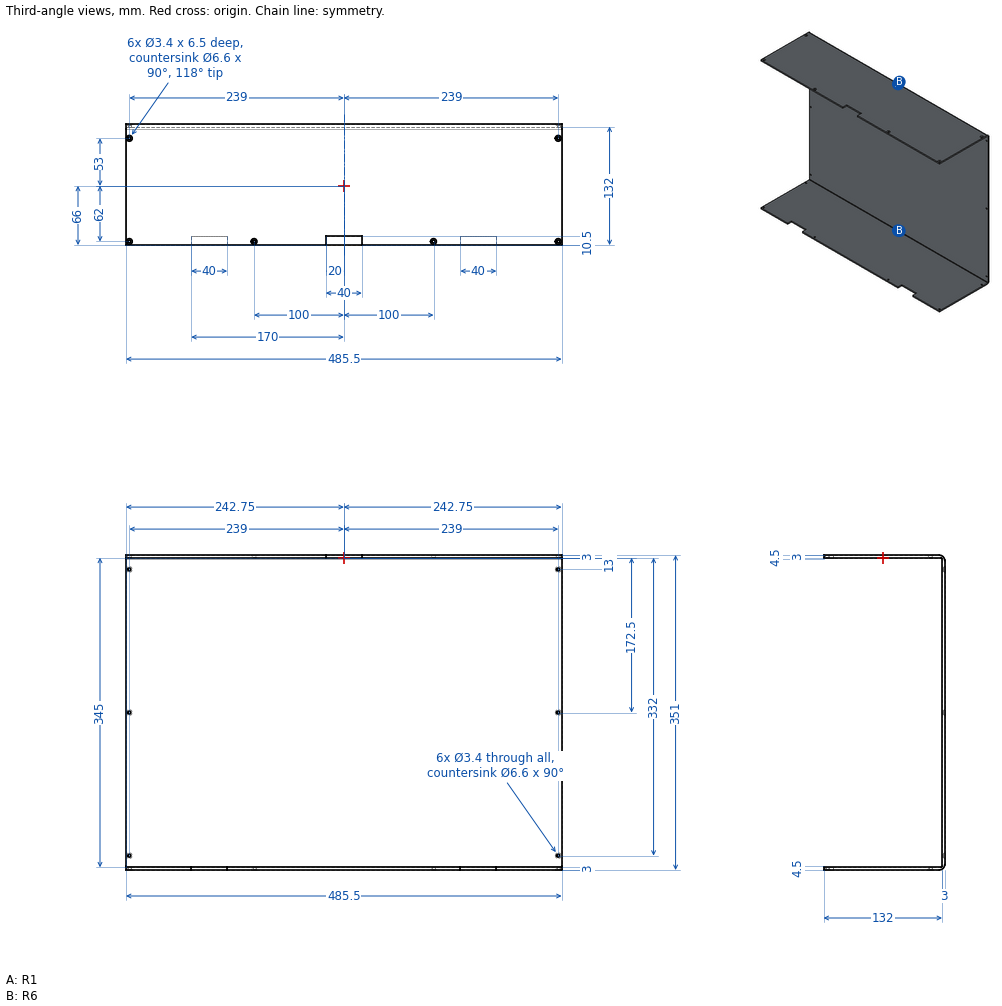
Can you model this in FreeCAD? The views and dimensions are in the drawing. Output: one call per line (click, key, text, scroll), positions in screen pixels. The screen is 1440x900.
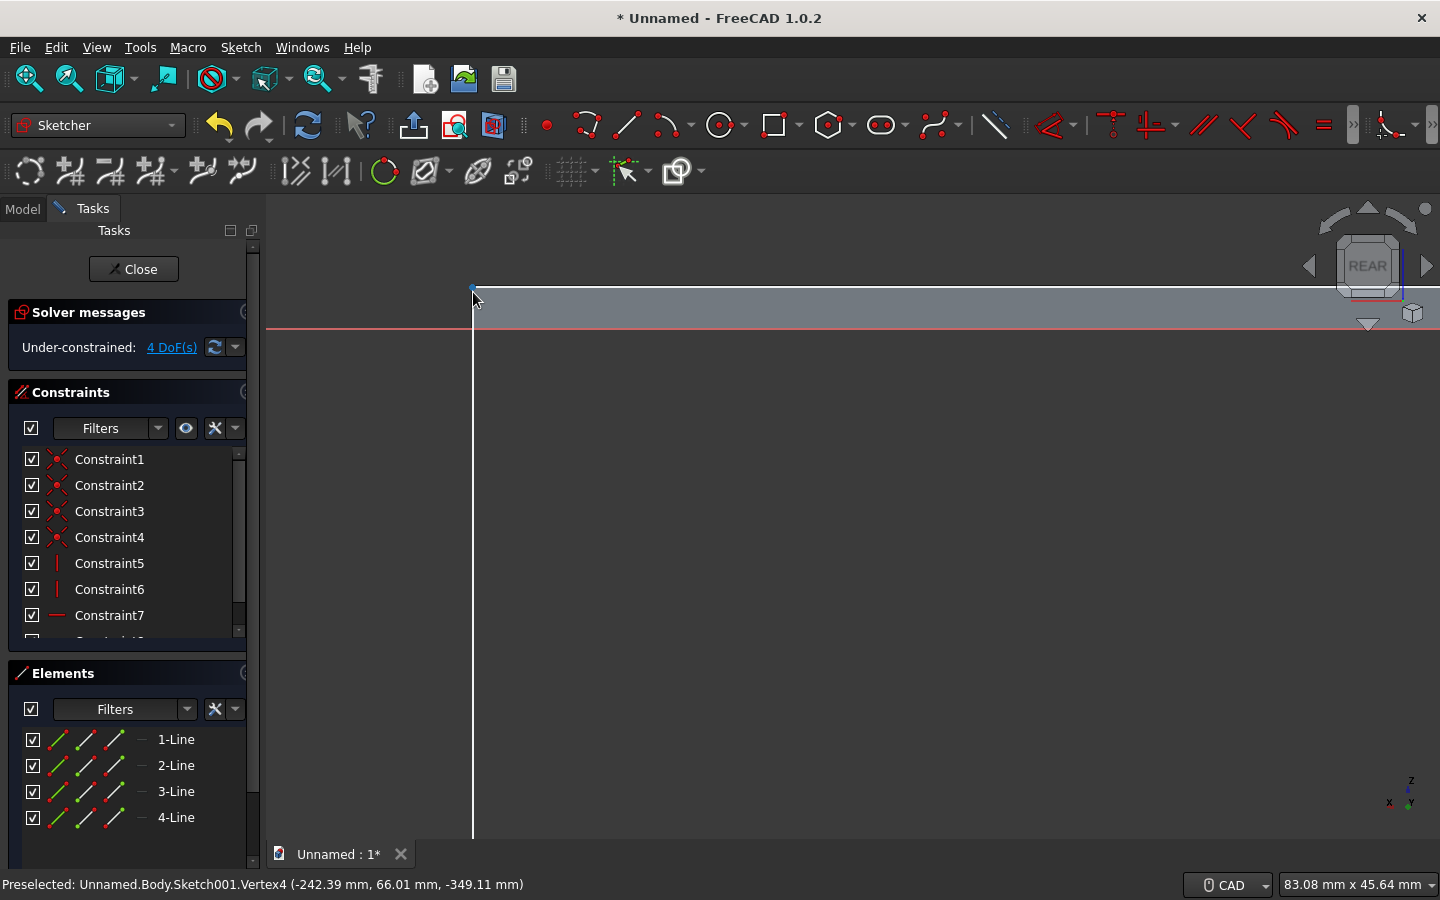
click(473, 287)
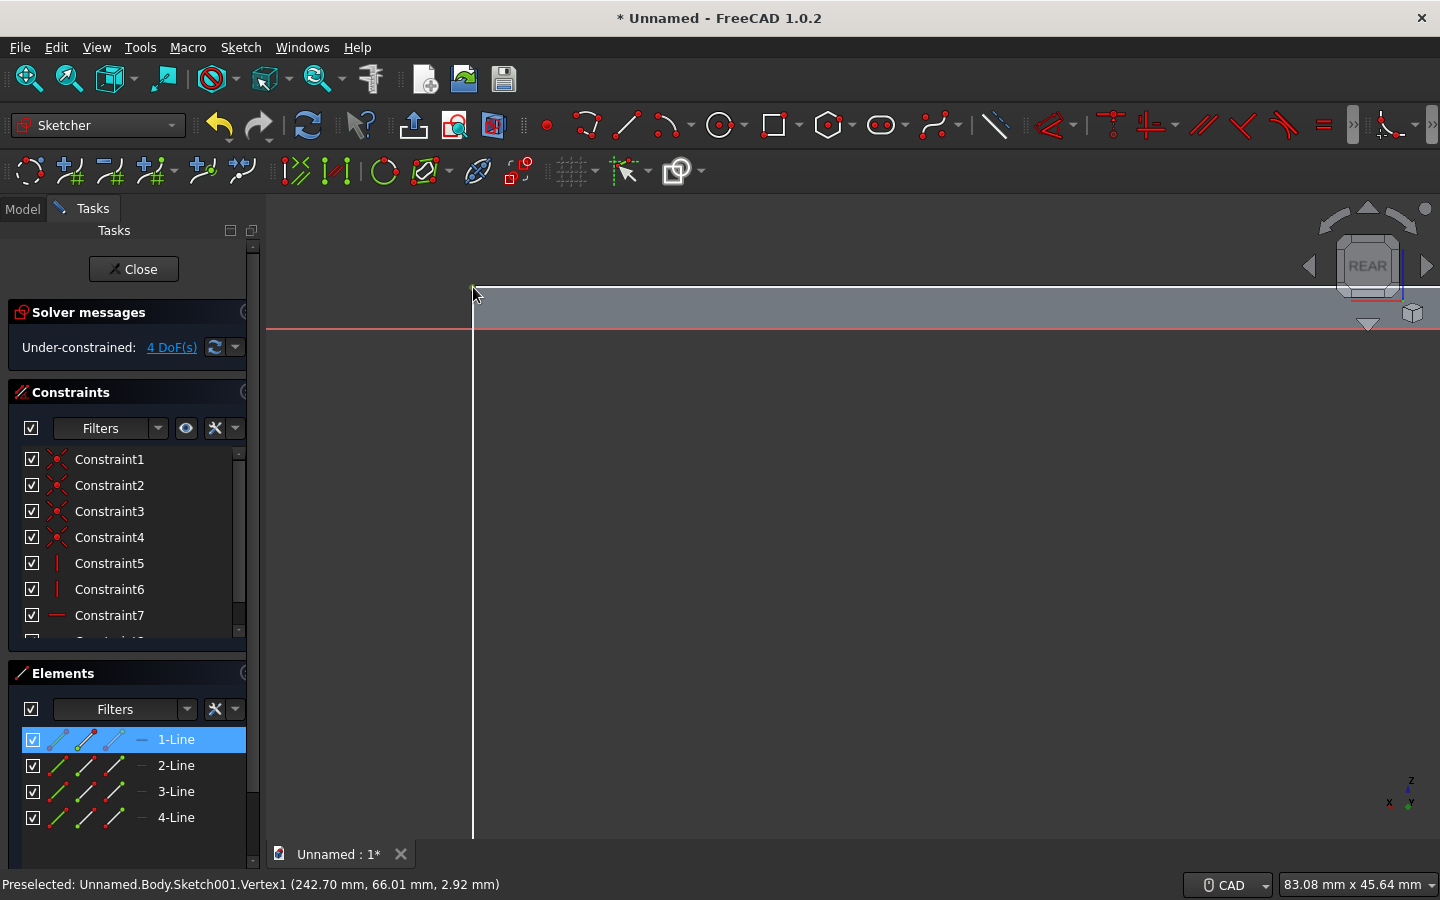
key(i)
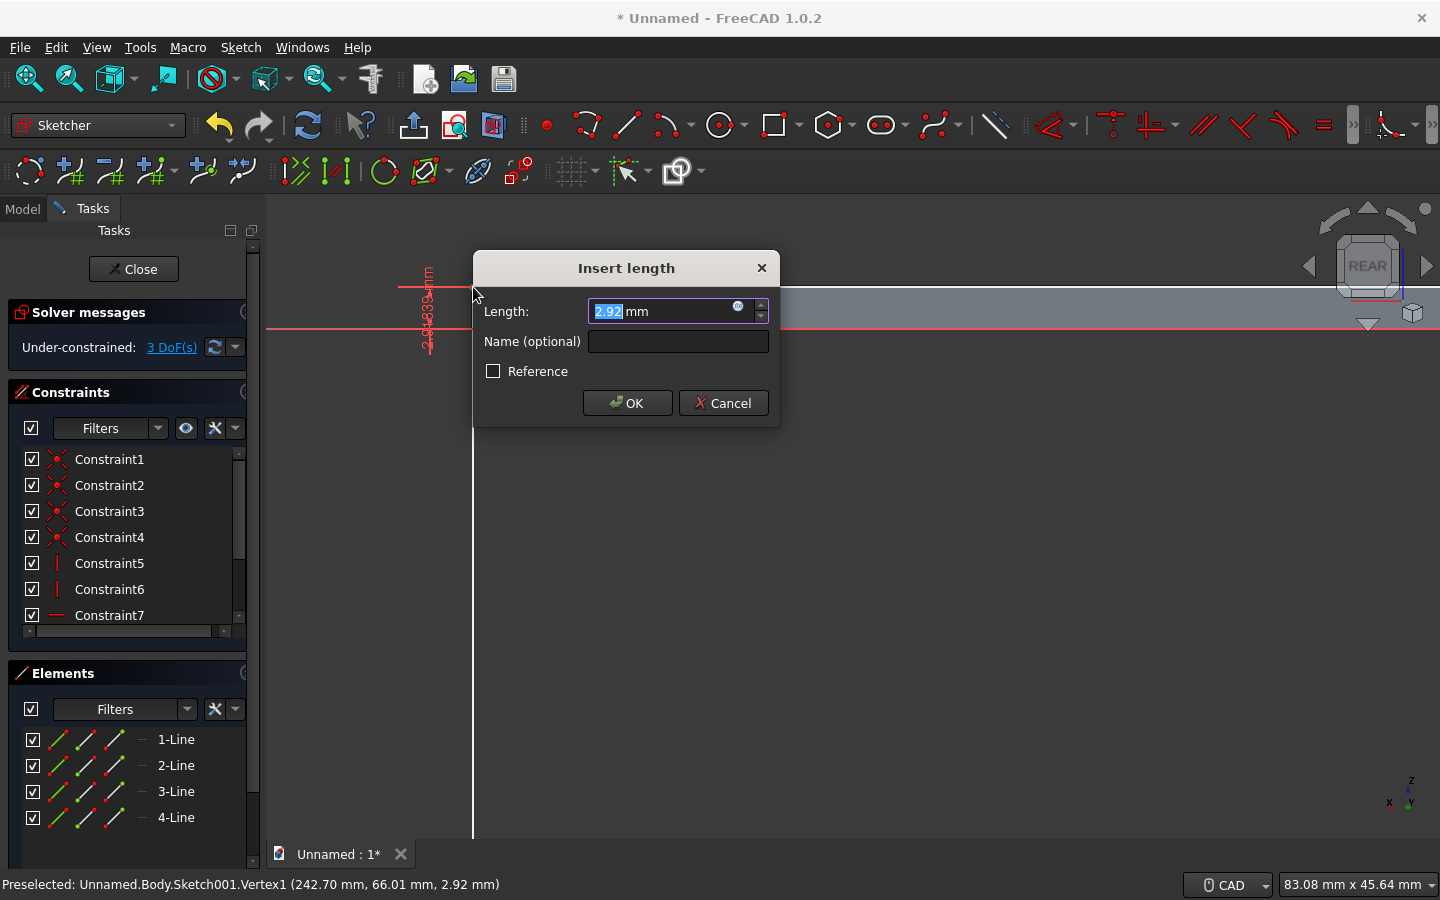
text(3)
key(Return)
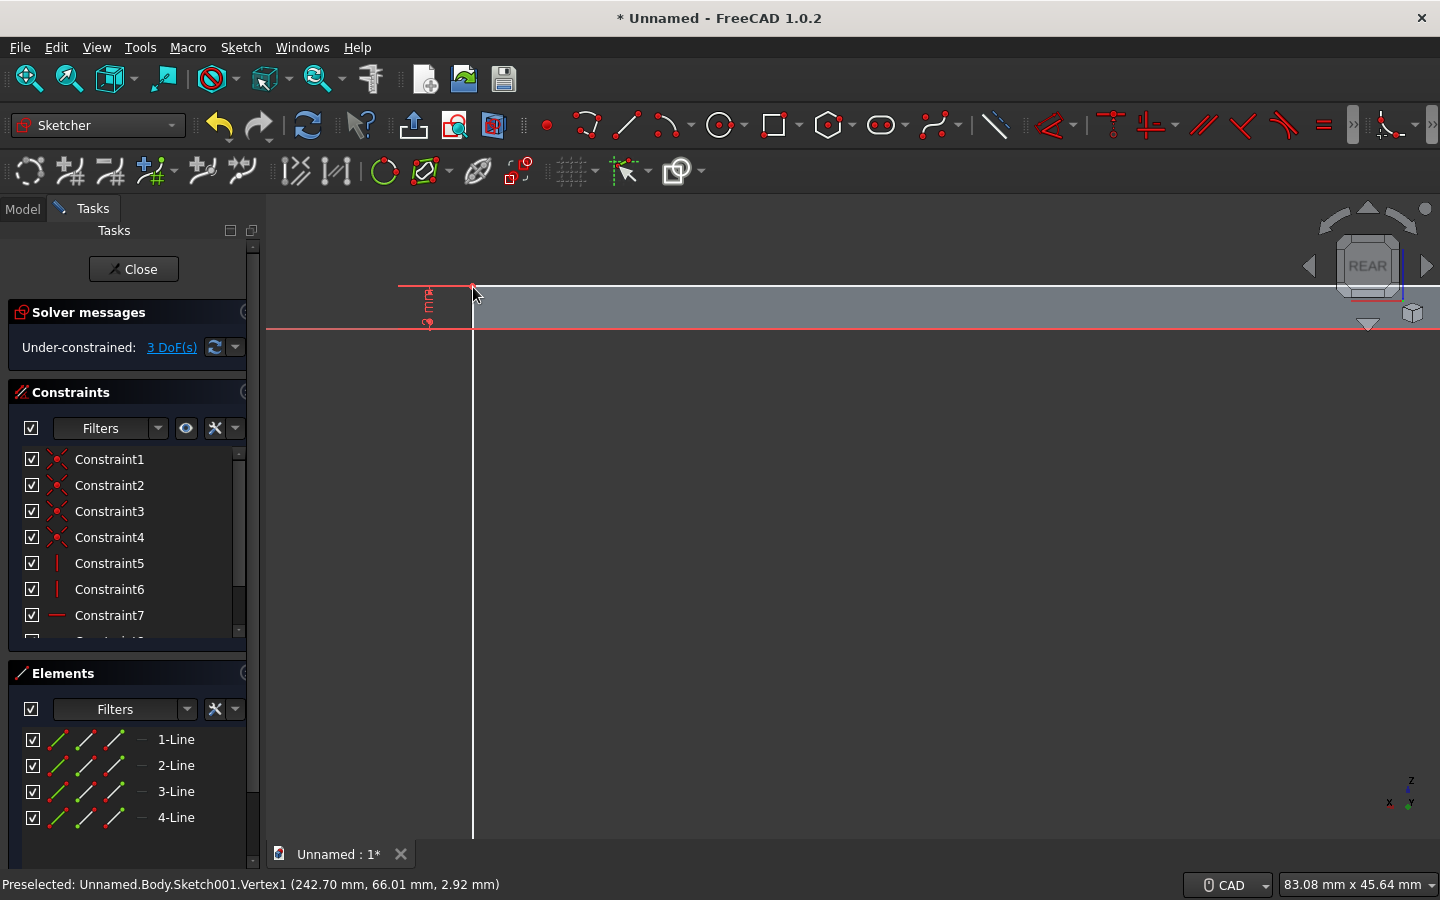
scroll(473, 292, down, 12)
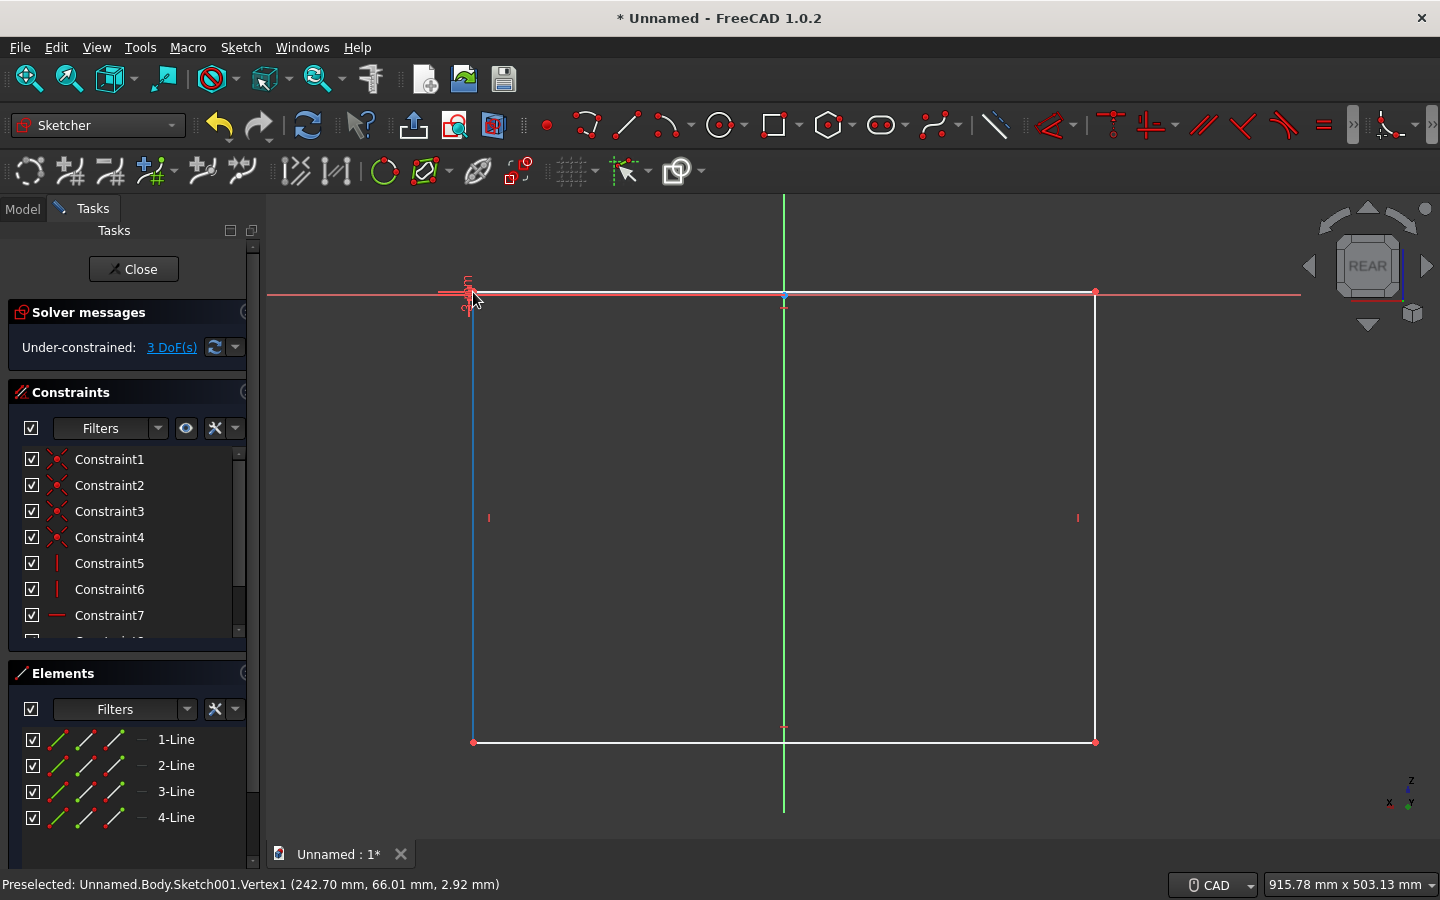
click(473, 427)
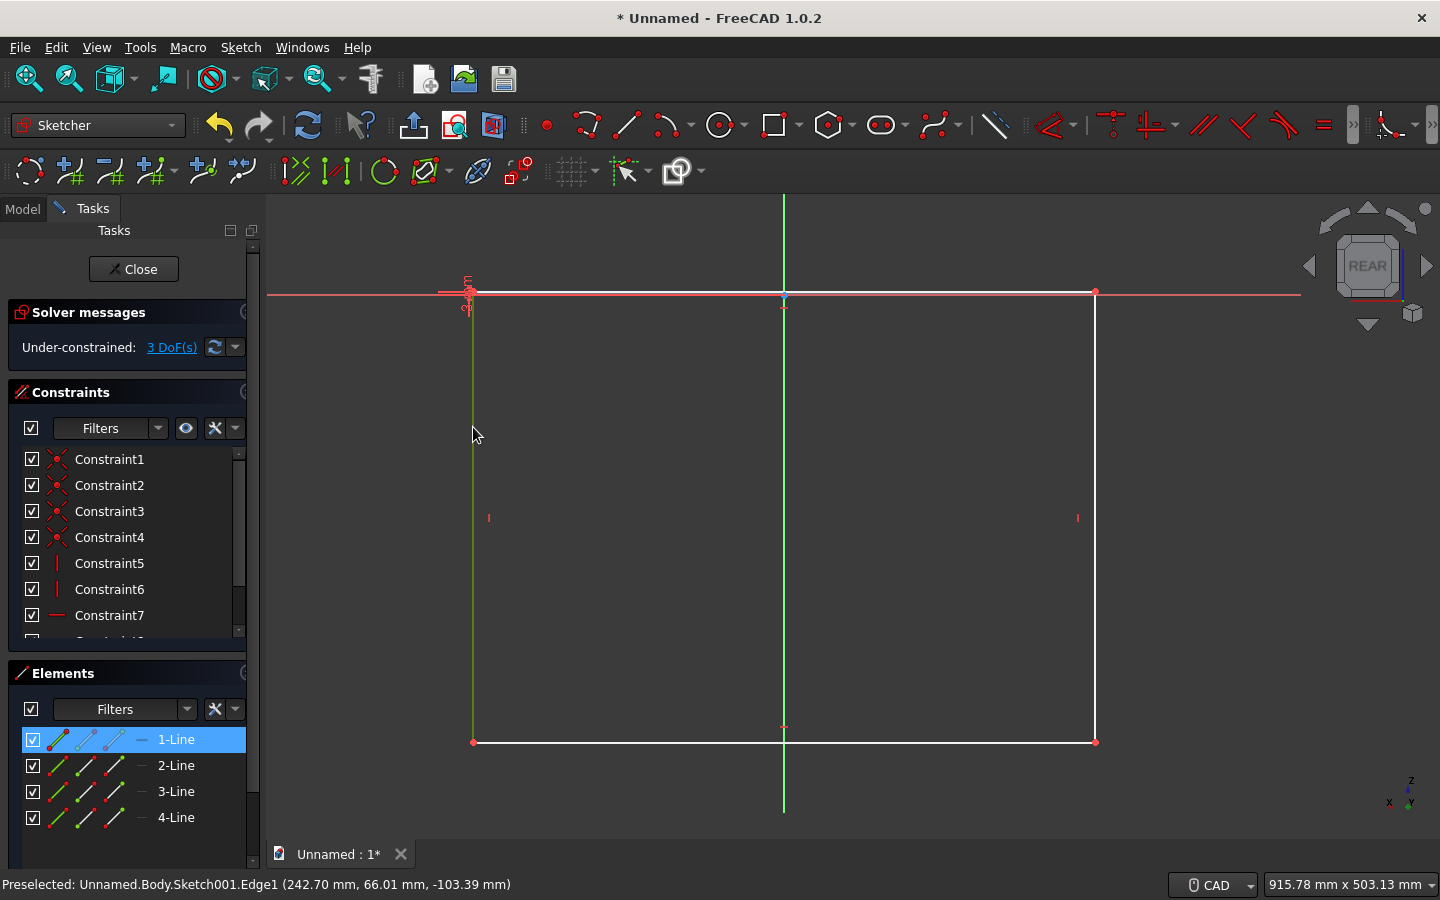
key(i)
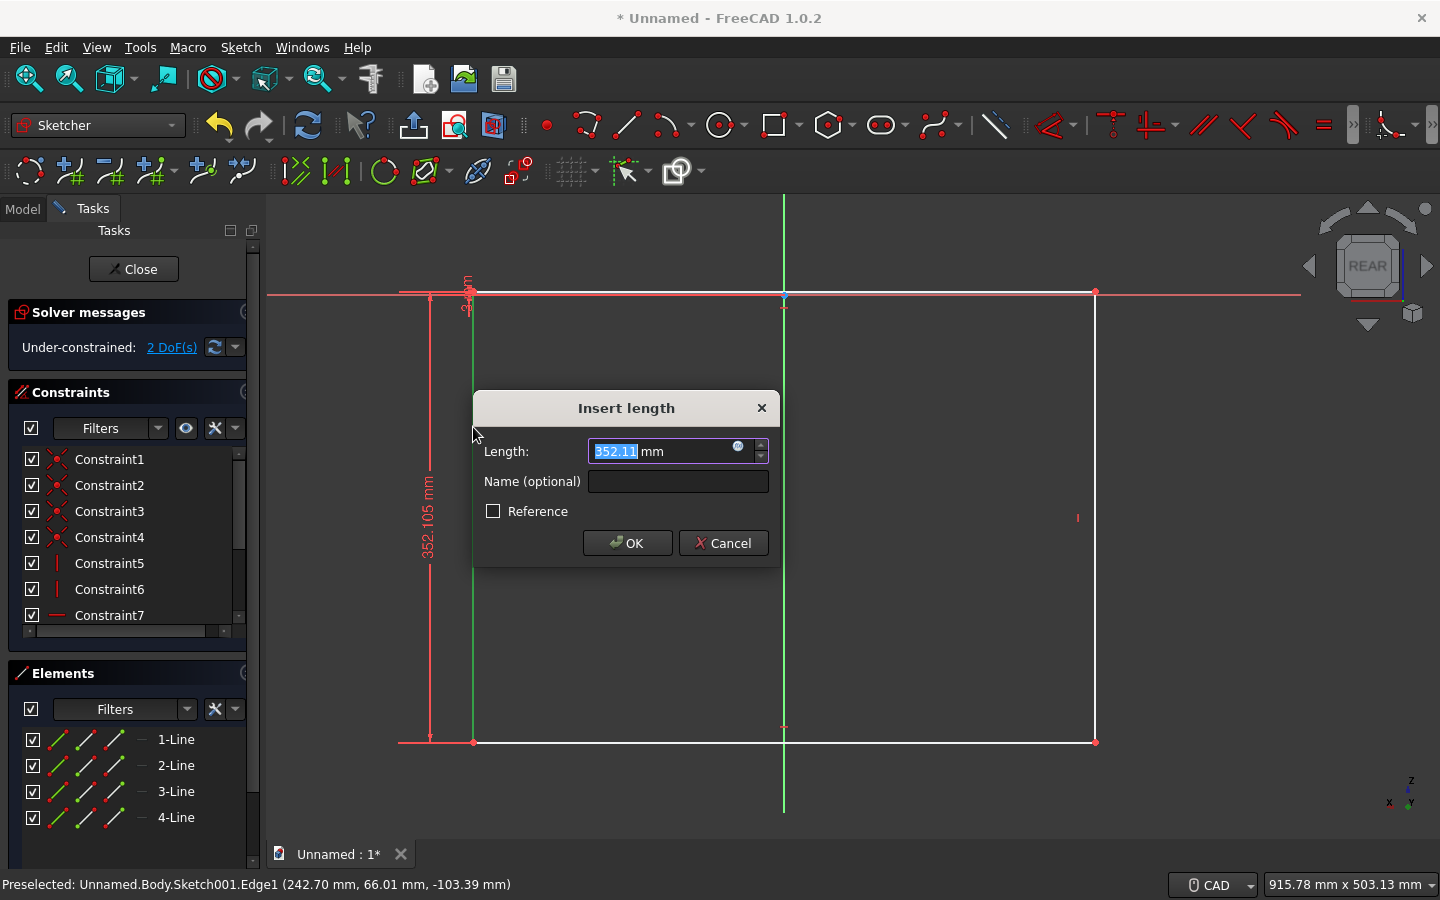
text(351)
key(Return)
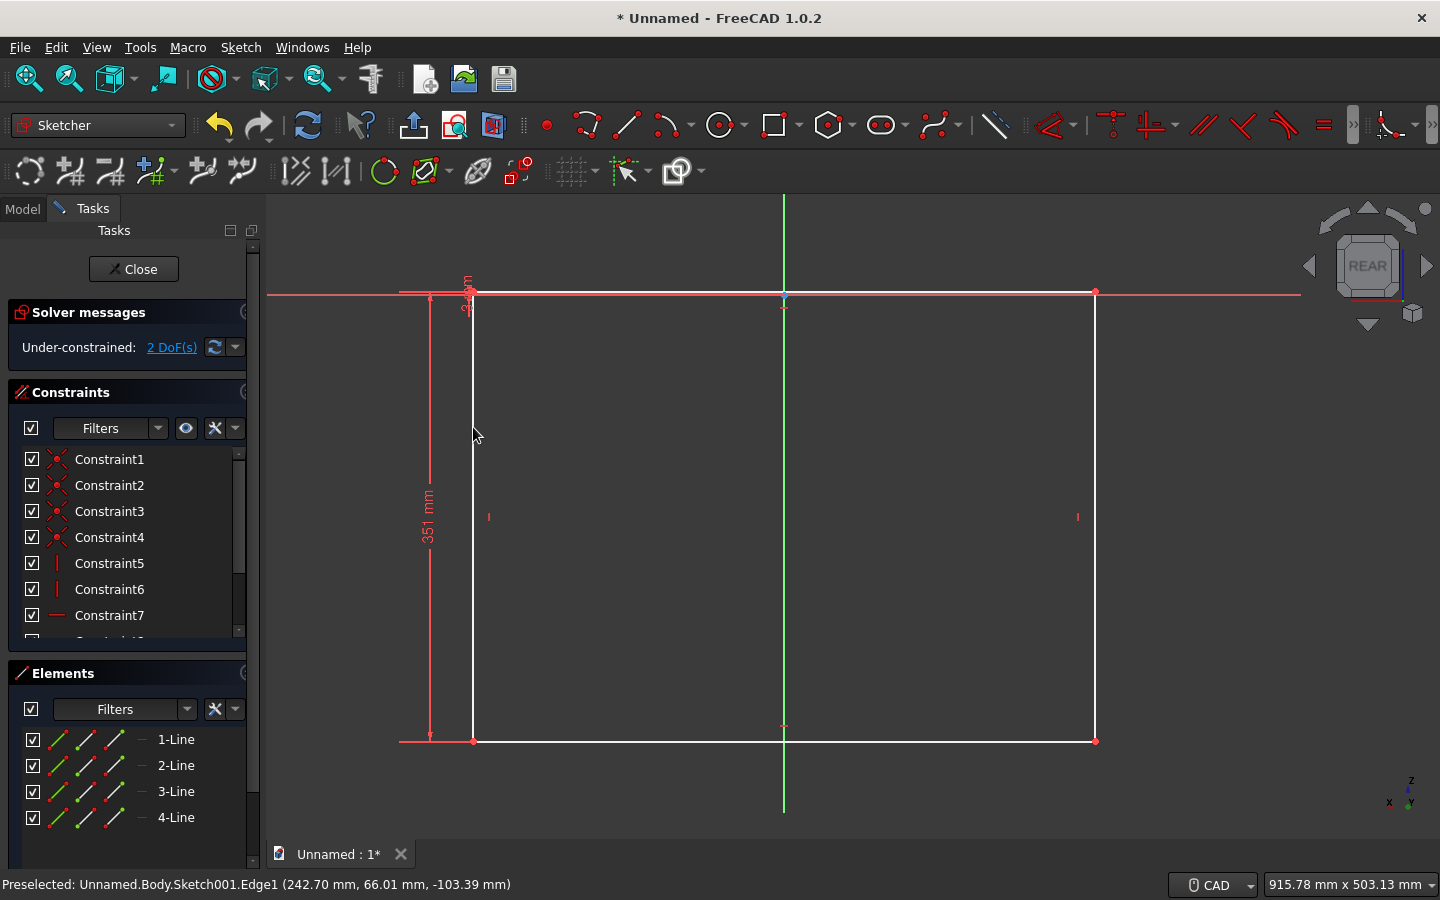
click(660, 742)